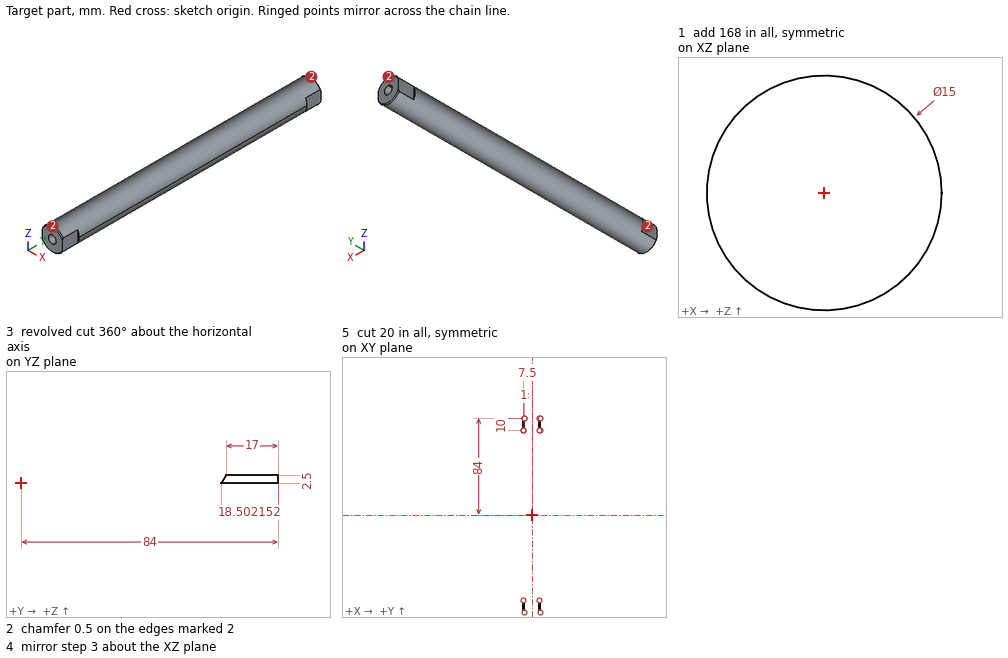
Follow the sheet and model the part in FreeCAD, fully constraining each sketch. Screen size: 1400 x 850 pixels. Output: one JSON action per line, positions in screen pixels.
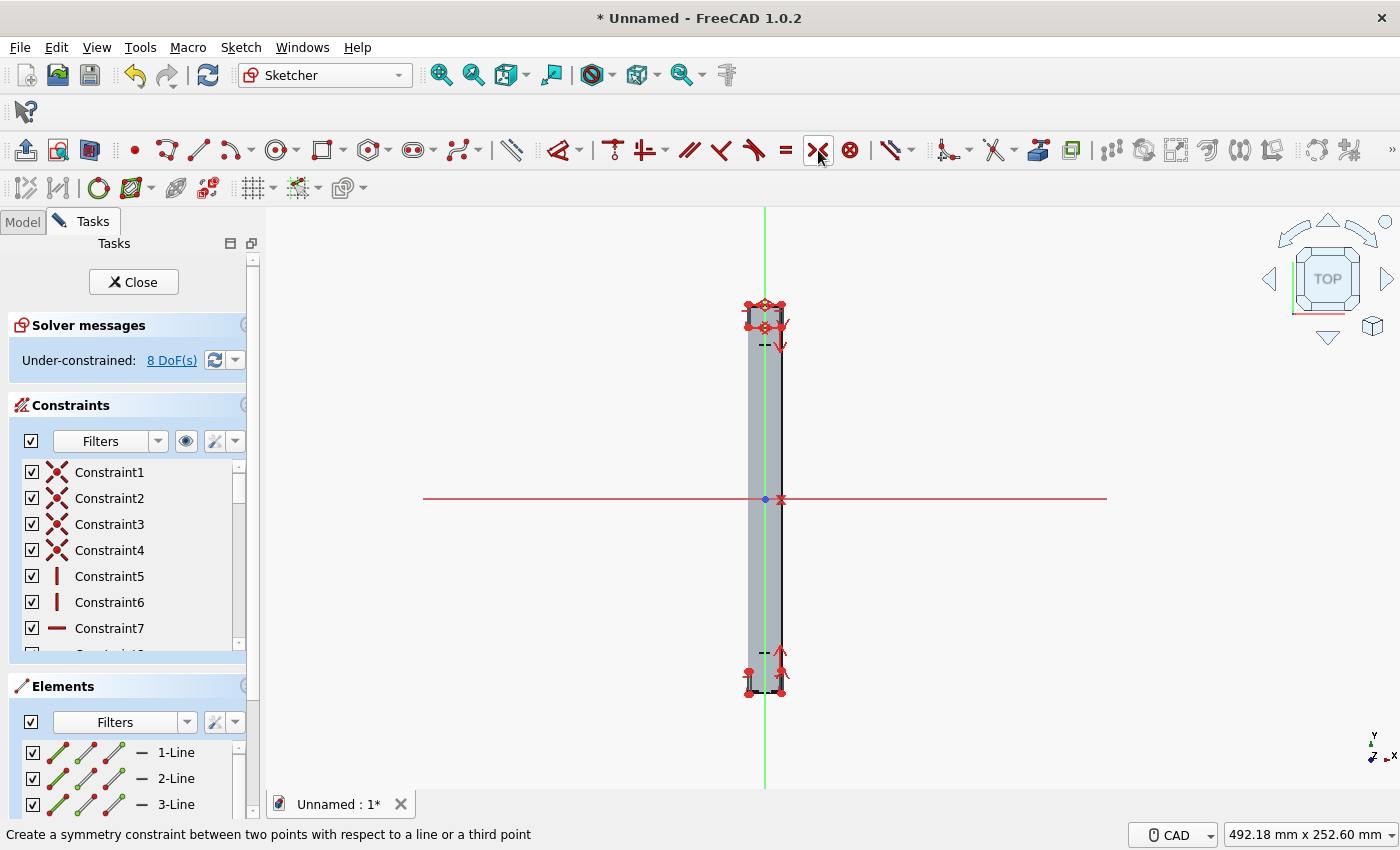
{"action": "scroll", "coordinate": [748, 328], "scroll_direction": "up", "scroll_amount": 9}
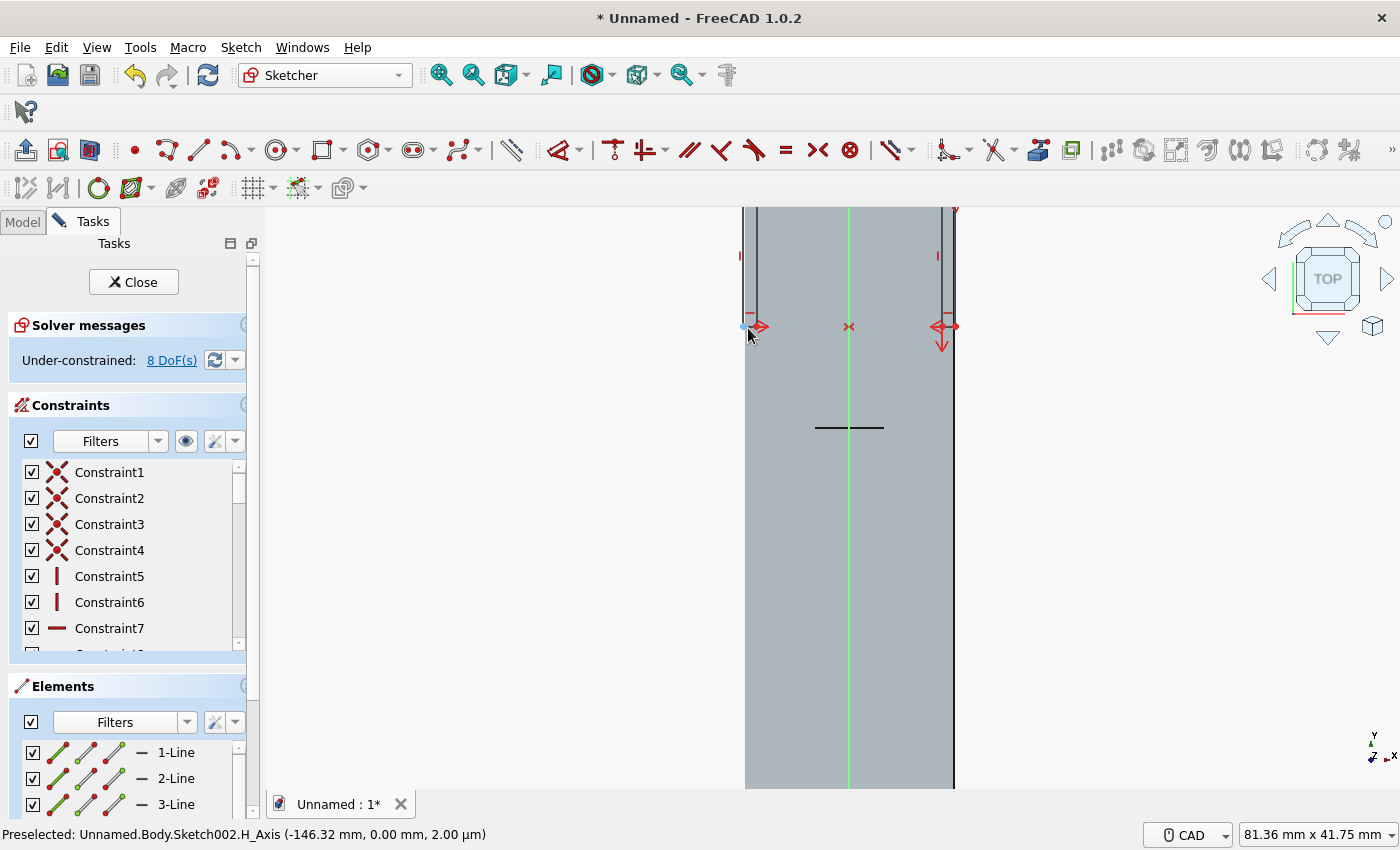
{"action": "left_click", "coordinate": [743, 327]}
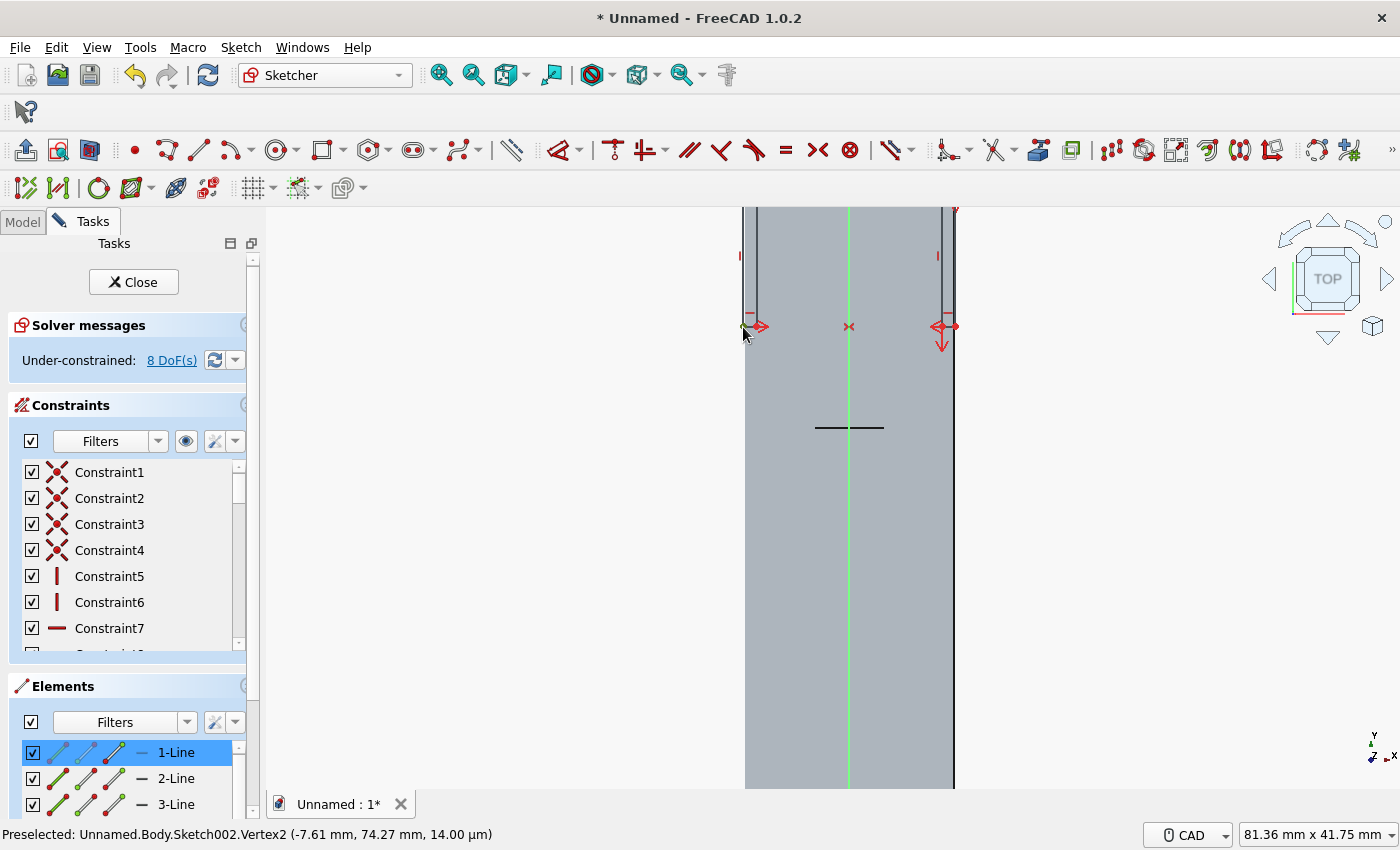
{"action": "scroll", "coordinate": [748, 327], "scroll_direction": "down", "scroll_amount": 9}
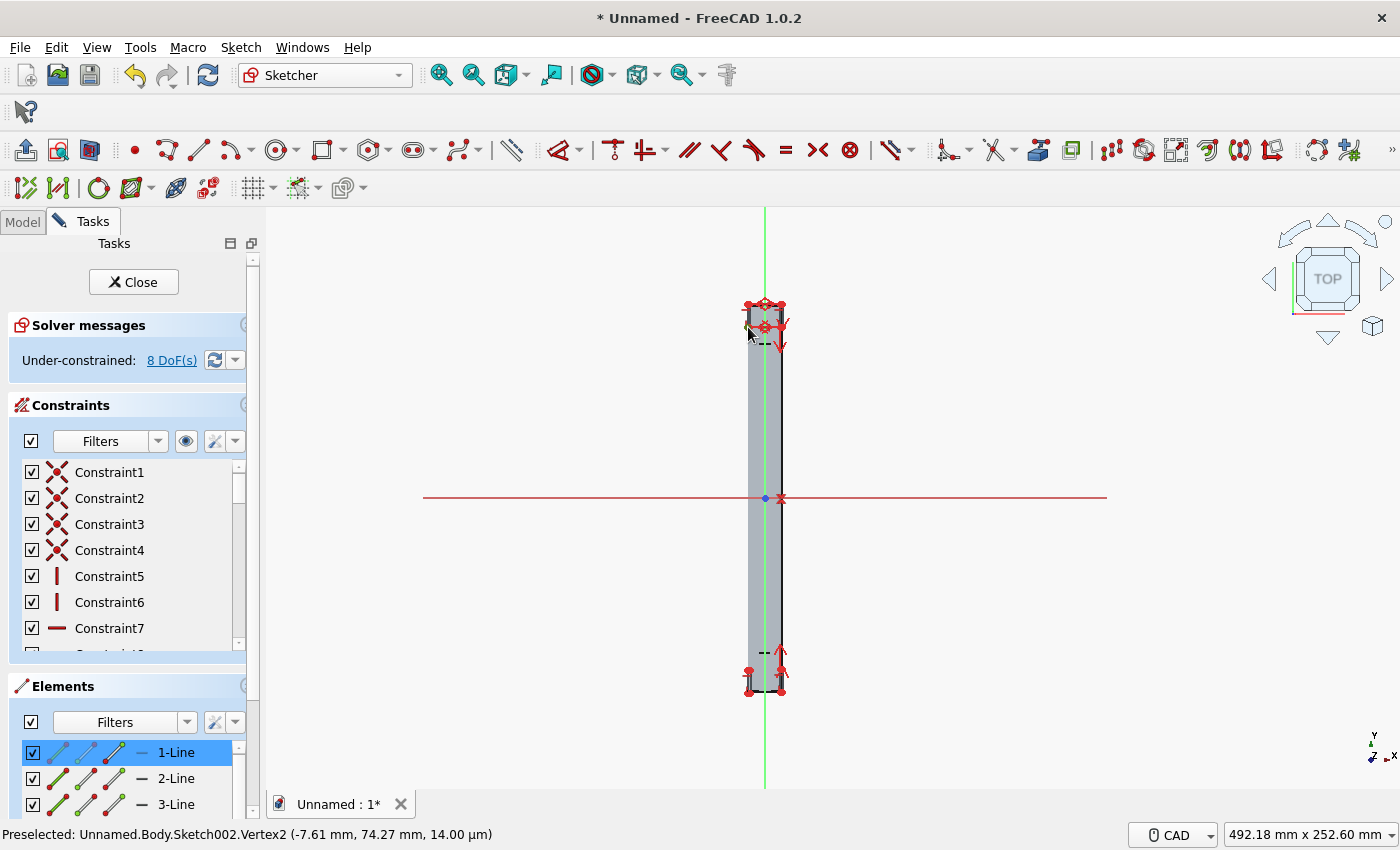
{"action": "scroll", "coordinate": [748, 670], "scroll_direction": "up", "scroll_amount": 8}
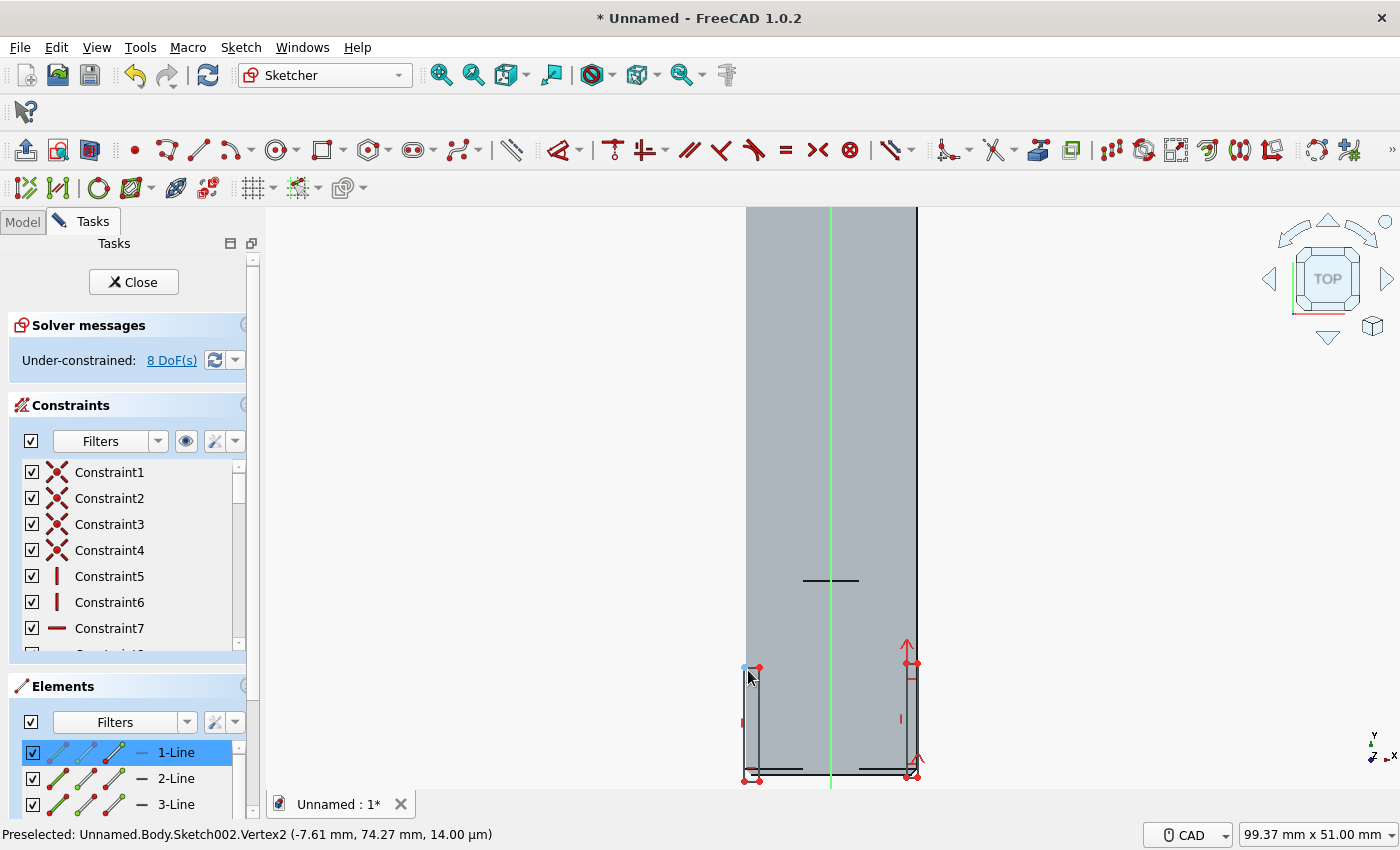
{"action": "left_click", "coordinate": [744, 668]}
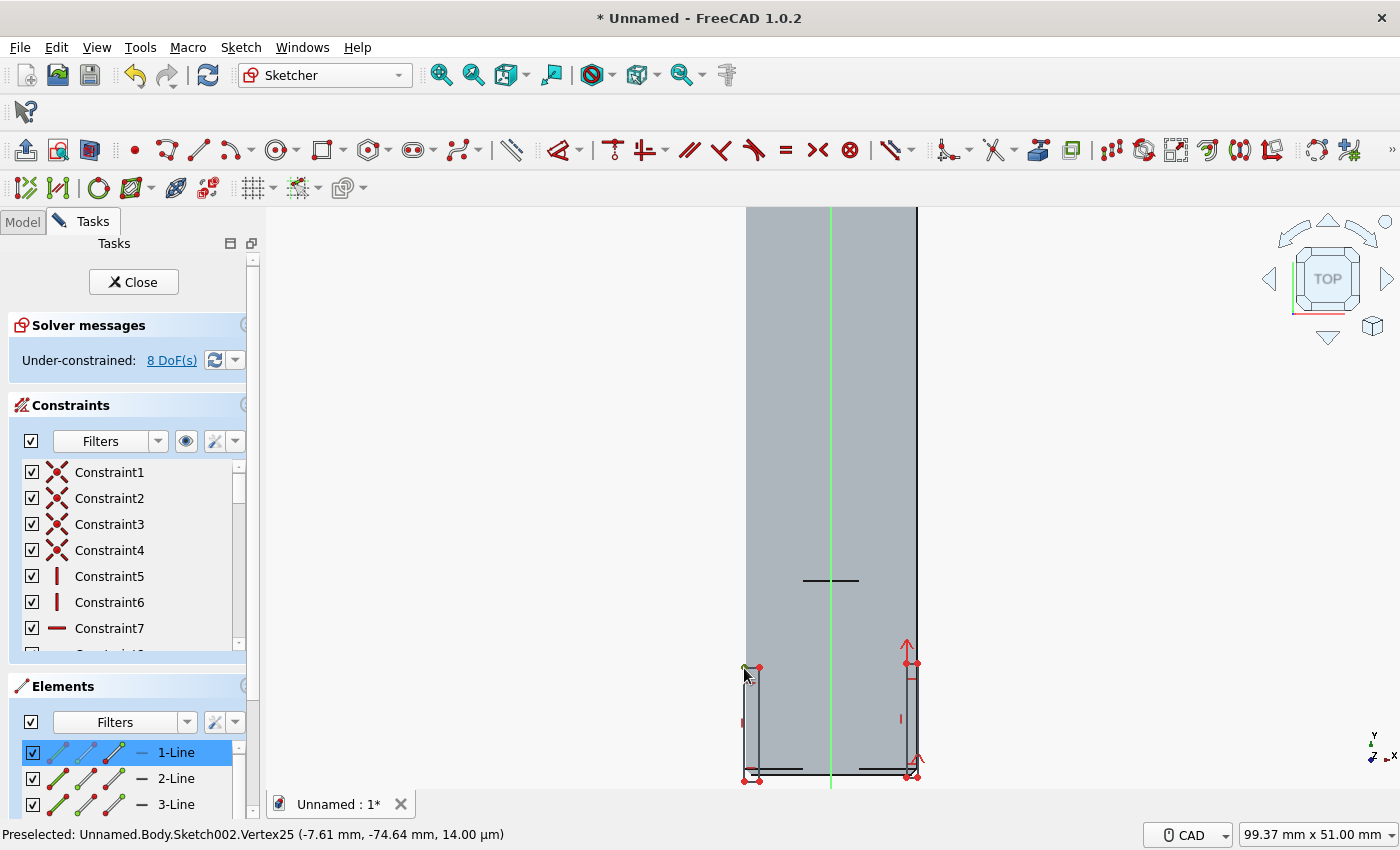
{"action": "scroll", "coordinate": [748, 670], "scroll_direction": "down", "scroll_amount": 8}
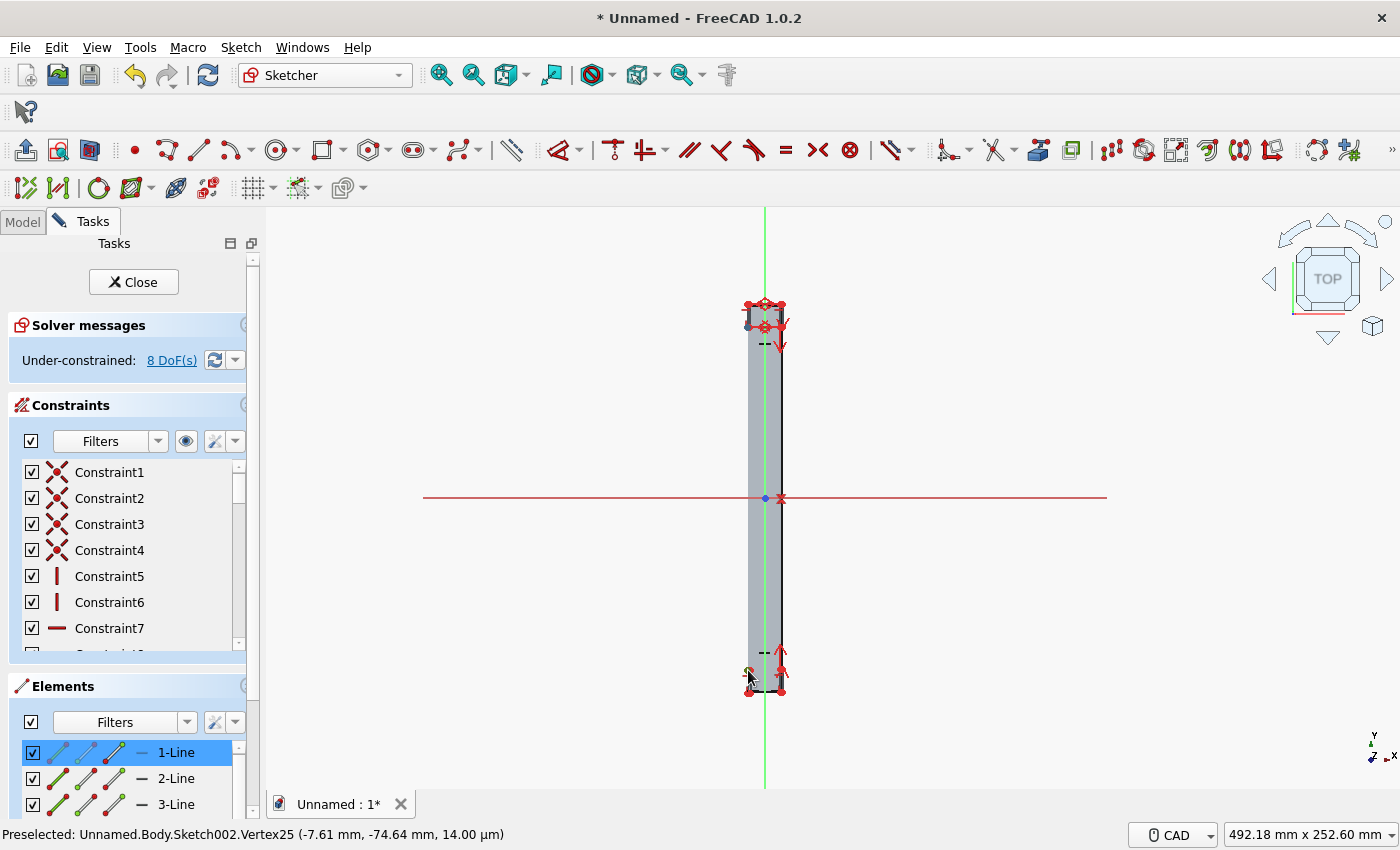
{"action": "left_click", "coordinate": [428, 498]}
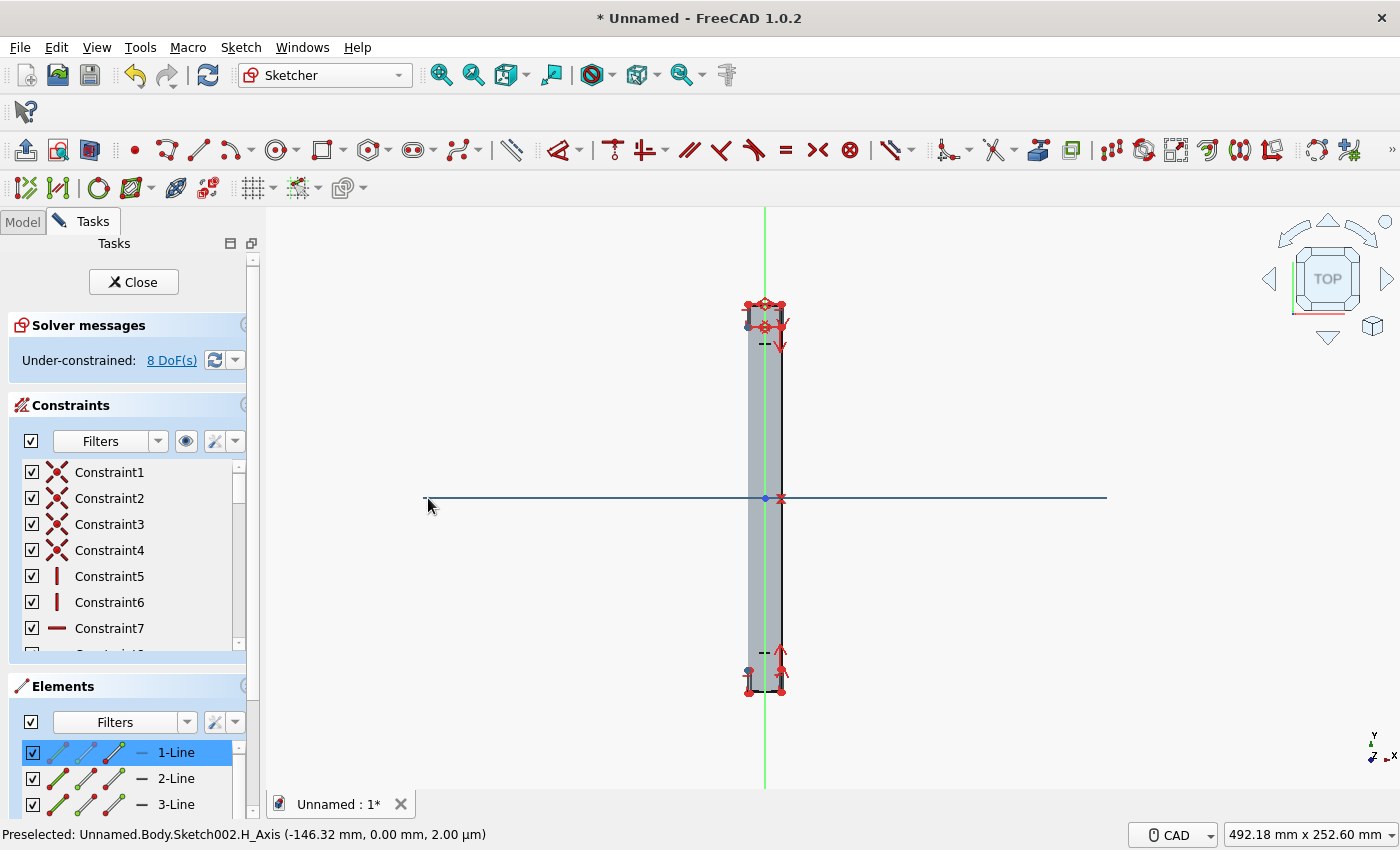
{"action": "left_click", "coordinate": [818, 150]}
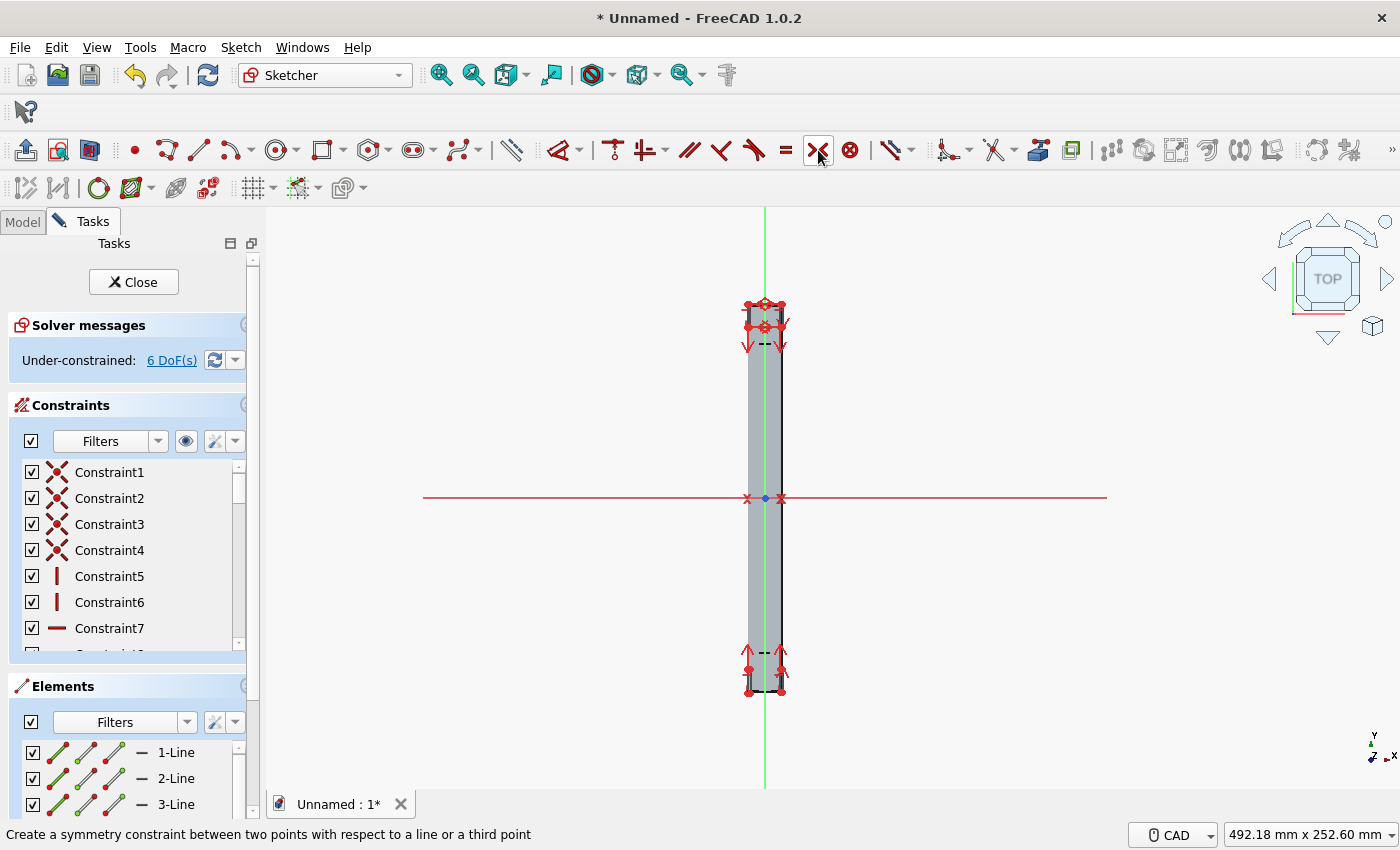
{"action": "scroll", "coordinate": [750, 304], "scroll_direction": "up", "scroll_amount": 9}